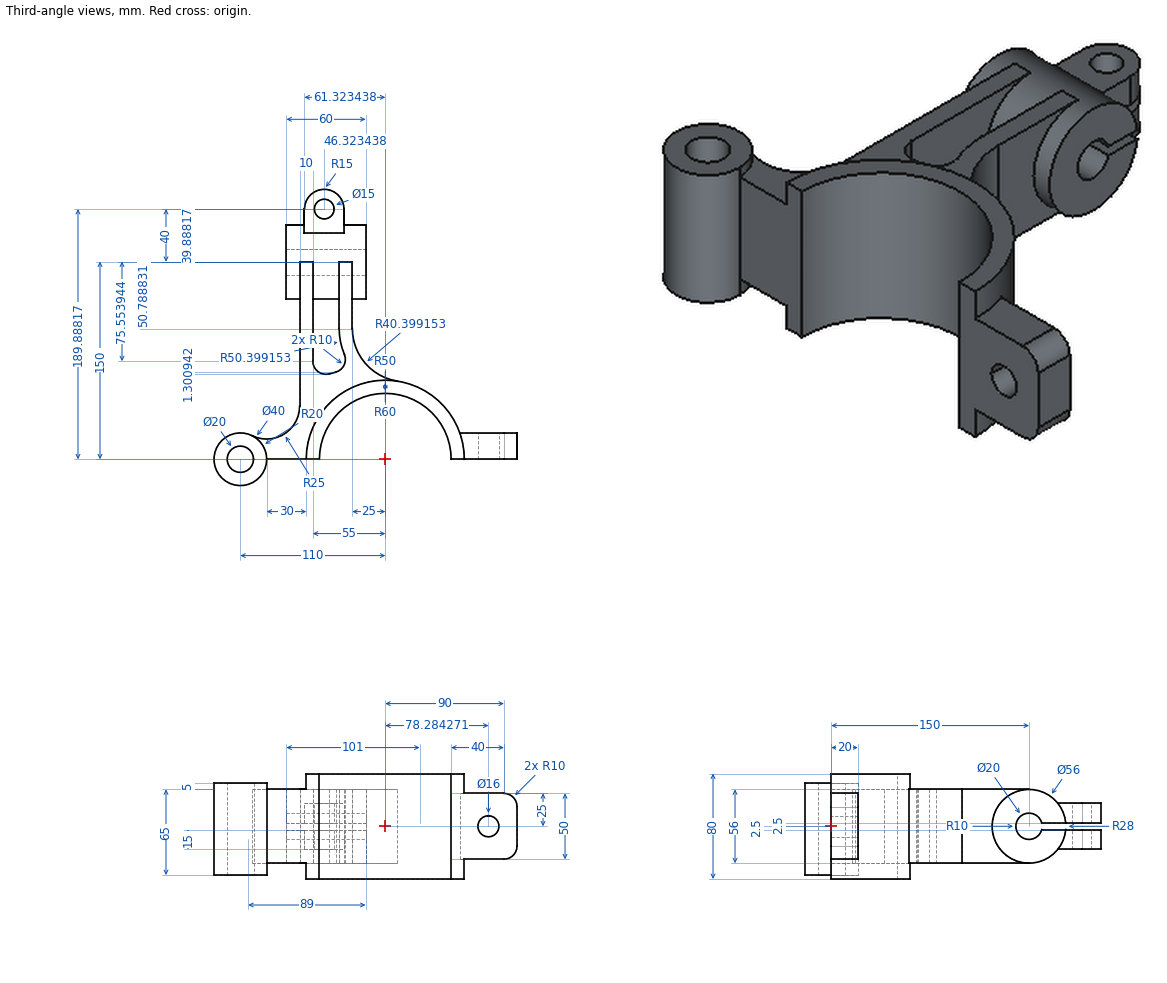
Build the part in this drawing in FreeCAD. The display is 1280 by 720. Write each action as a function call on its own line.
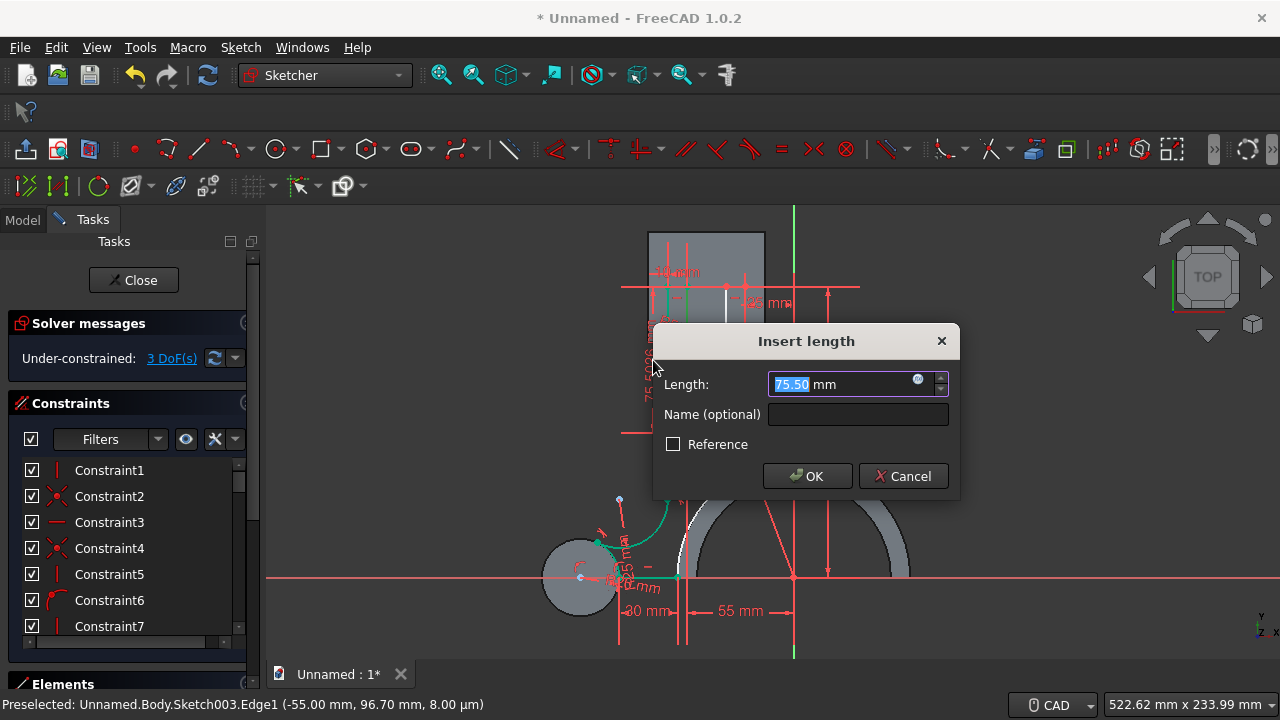
text(75.553944)
key(Return)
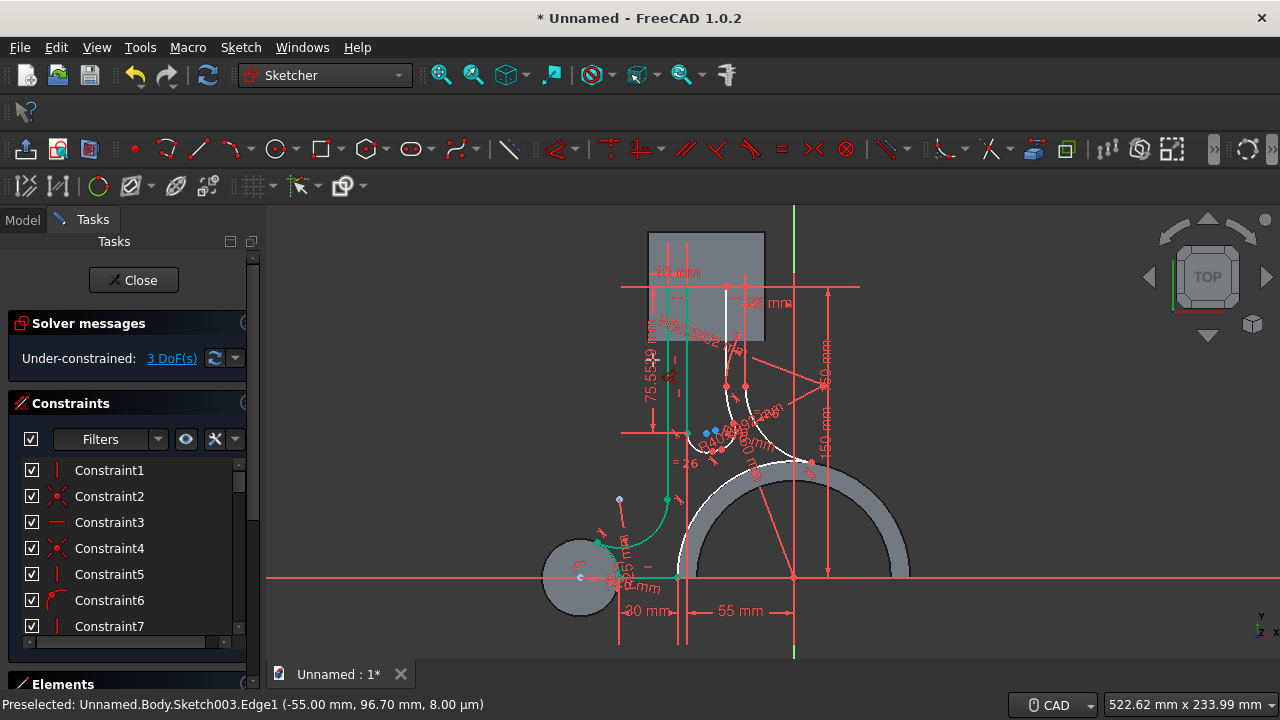
click(745, 357)
click(779, 337)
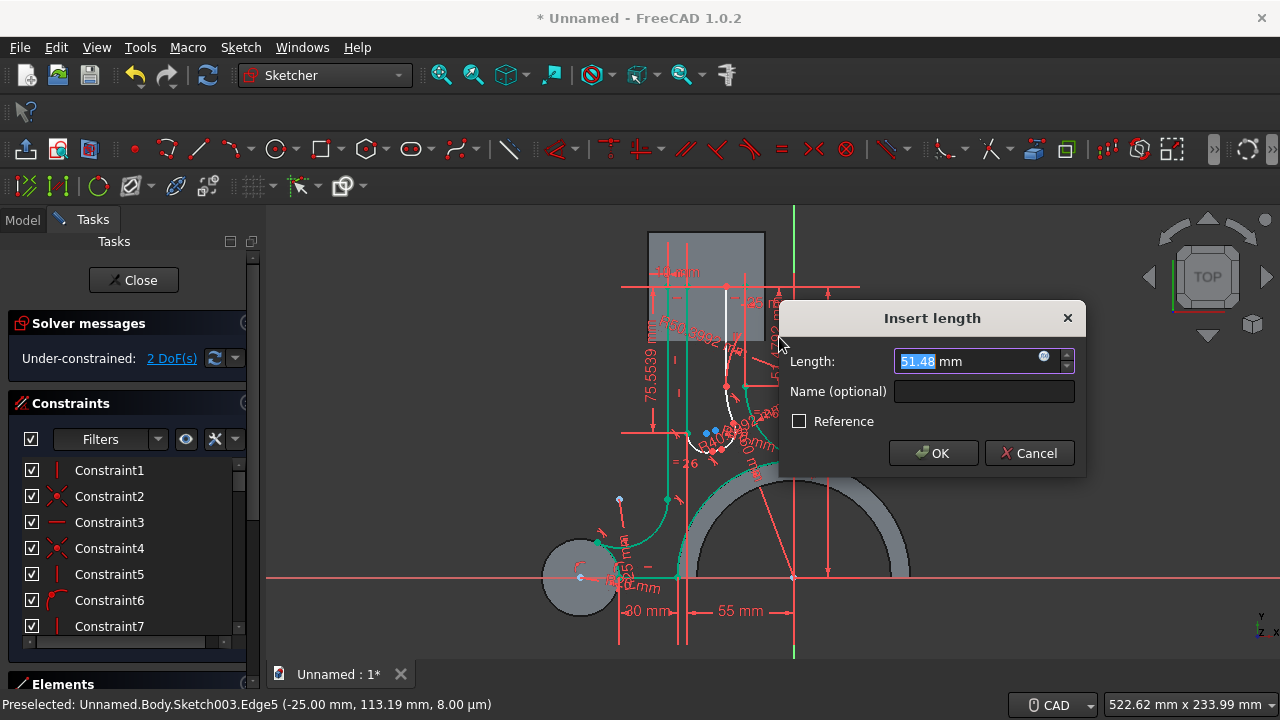
text(50.788831)
key(Return)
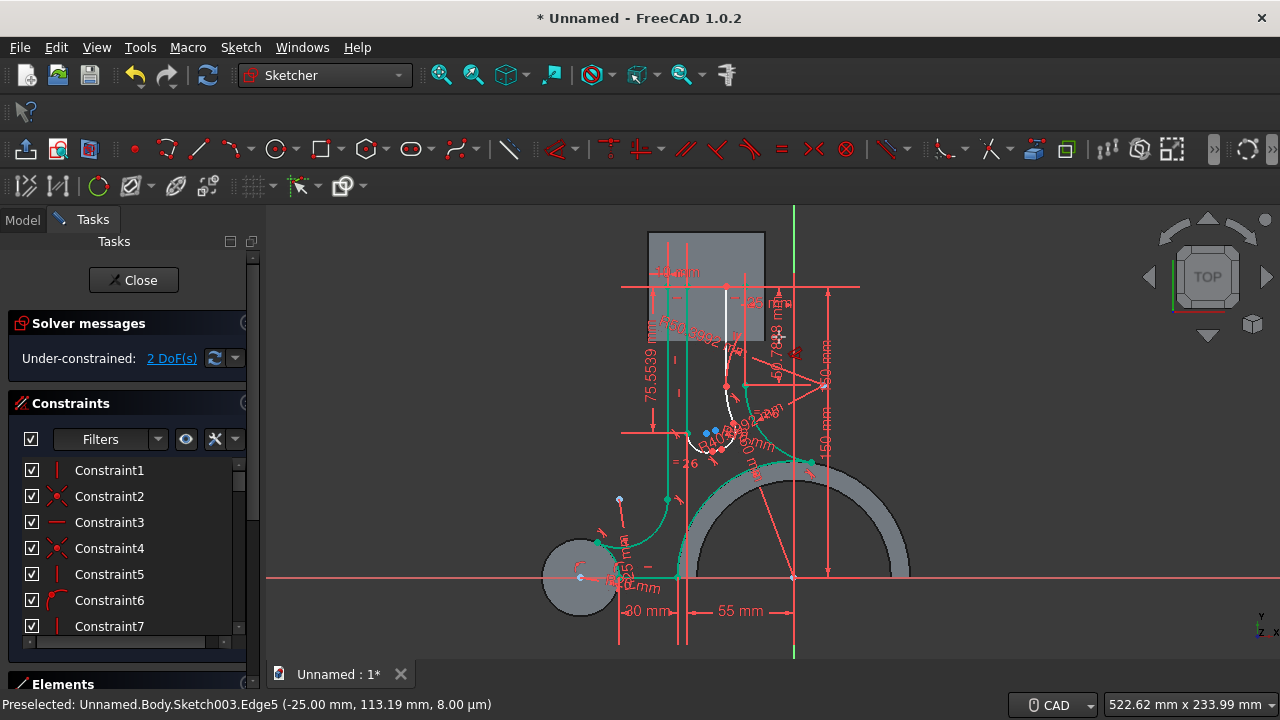
click(726, 317)
click(644, 314)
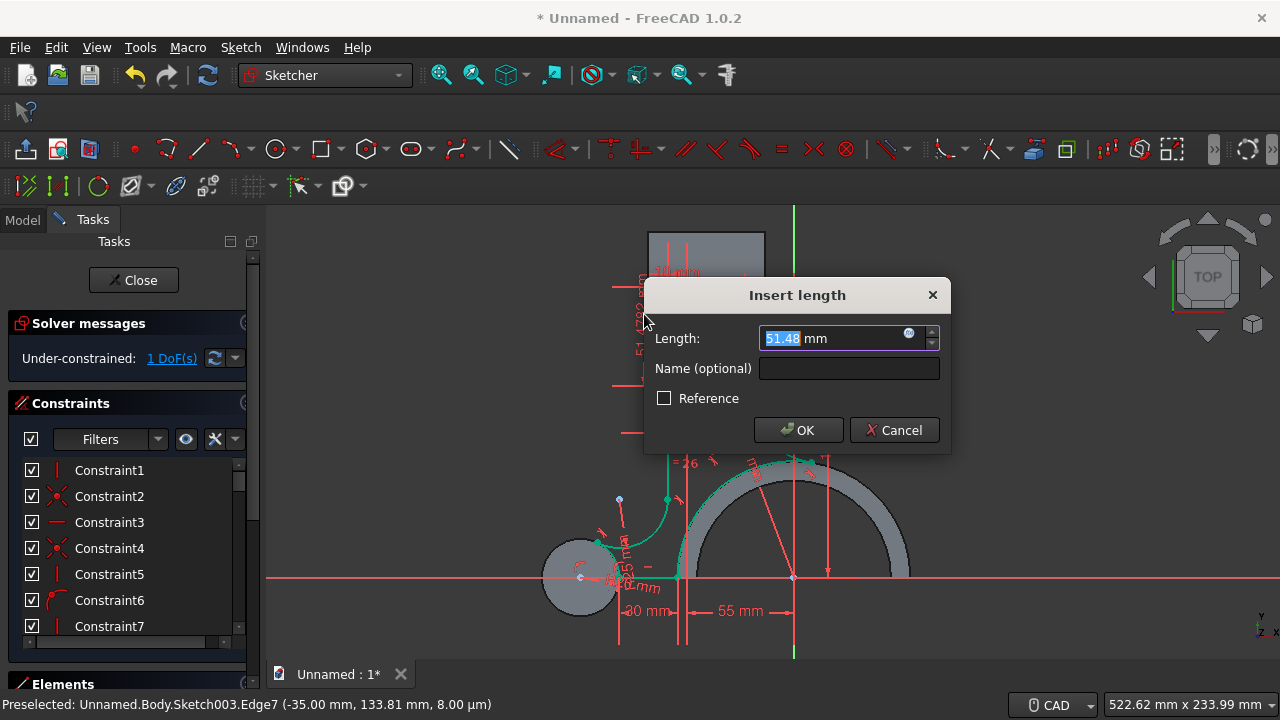
text(50.788831)
key(Return)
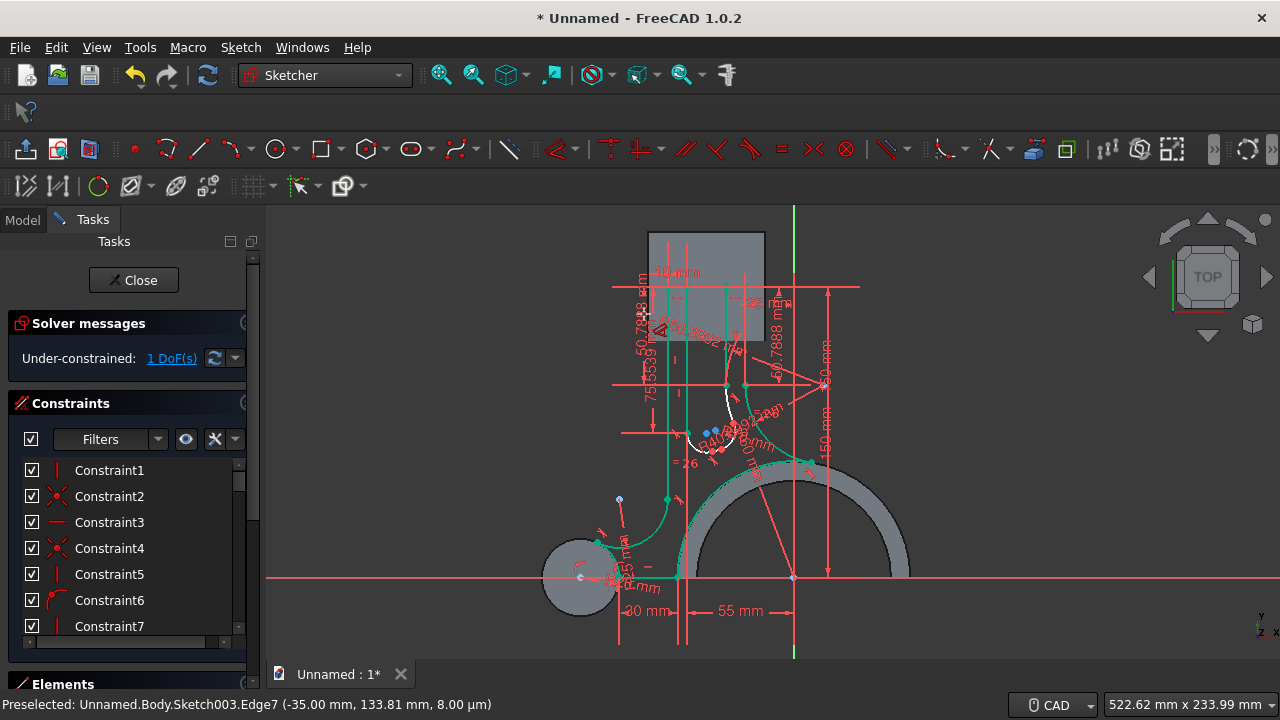
scroll(717, 450, up, 14)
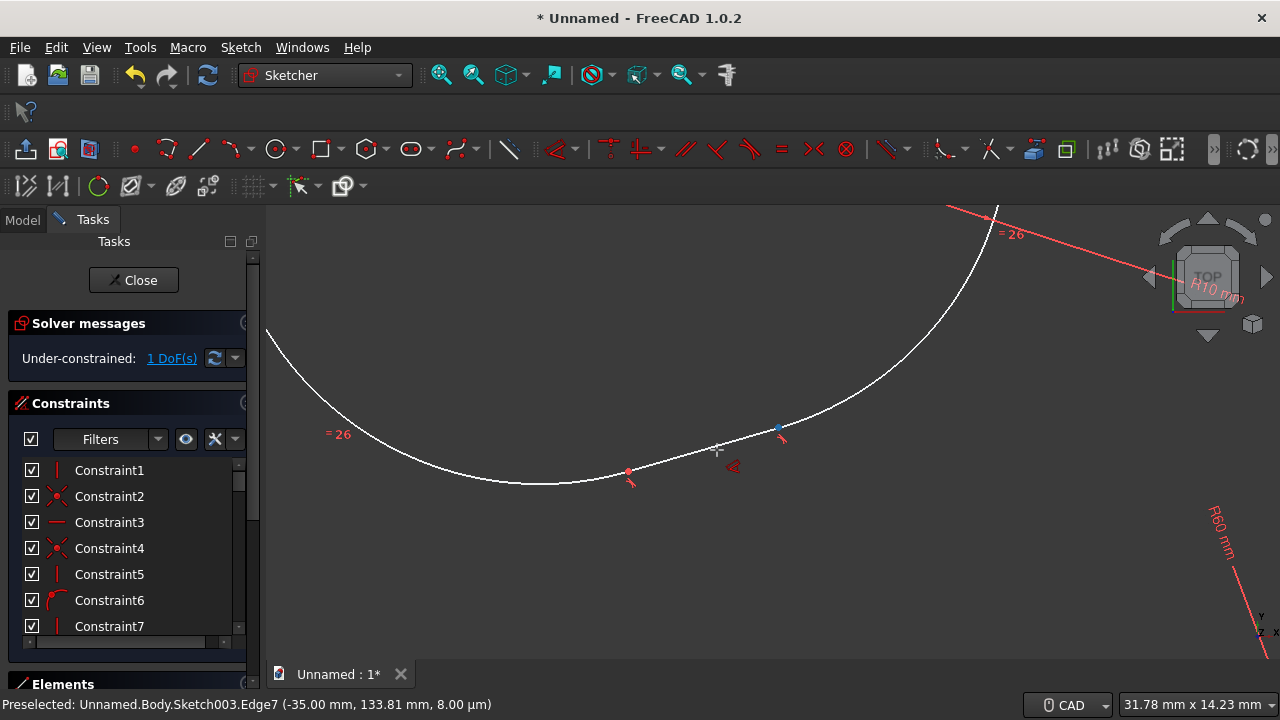
click(704, 450)
click(813, 450)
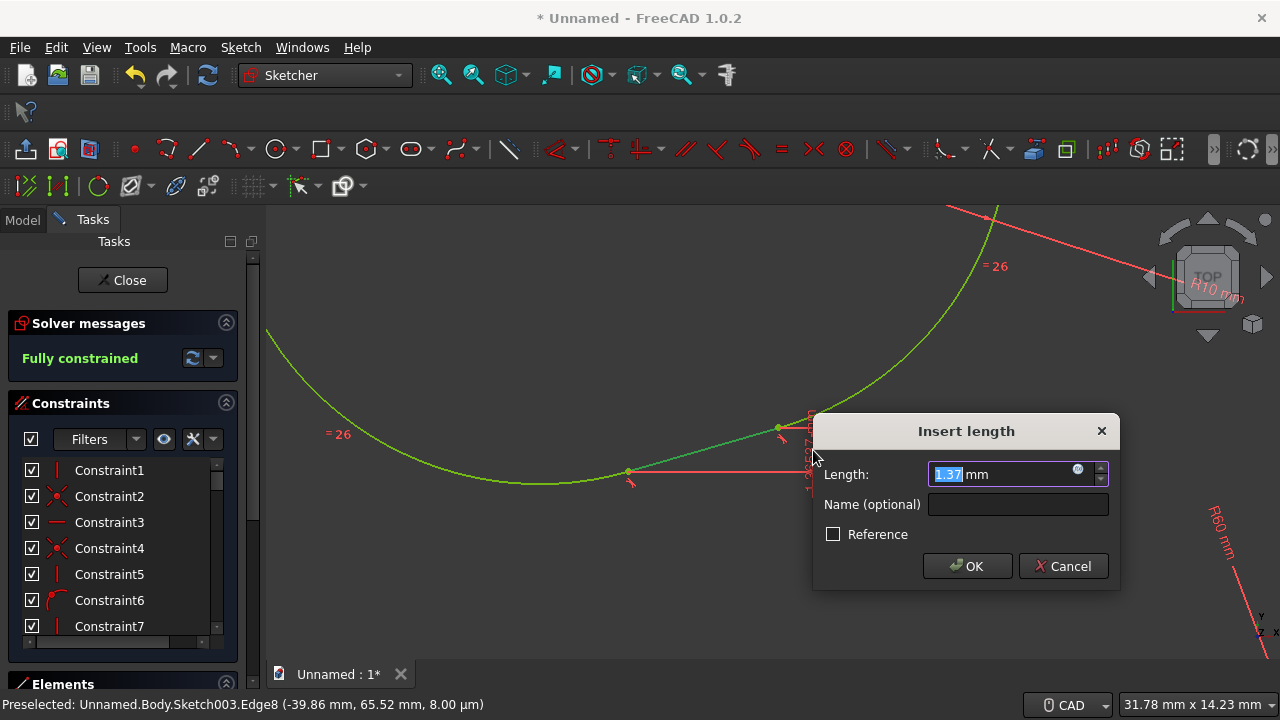
text(1.300942)
key(Return)
key(Escape)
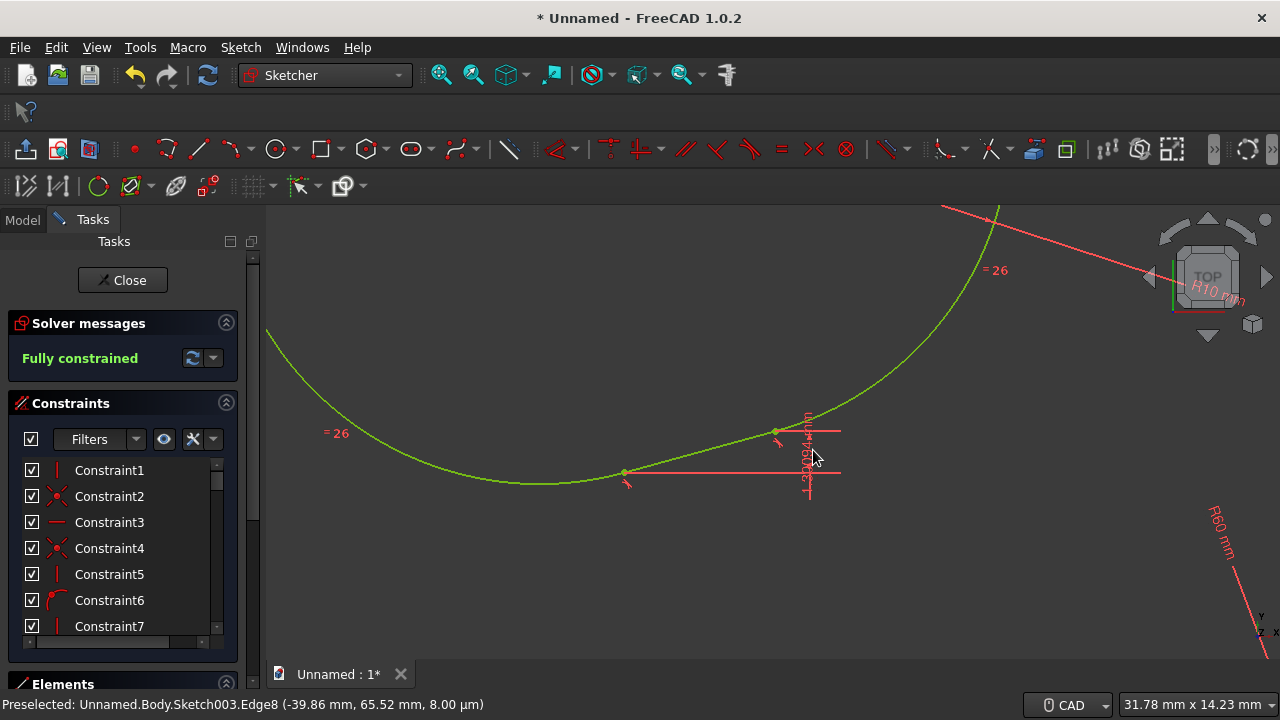
click(123, 280)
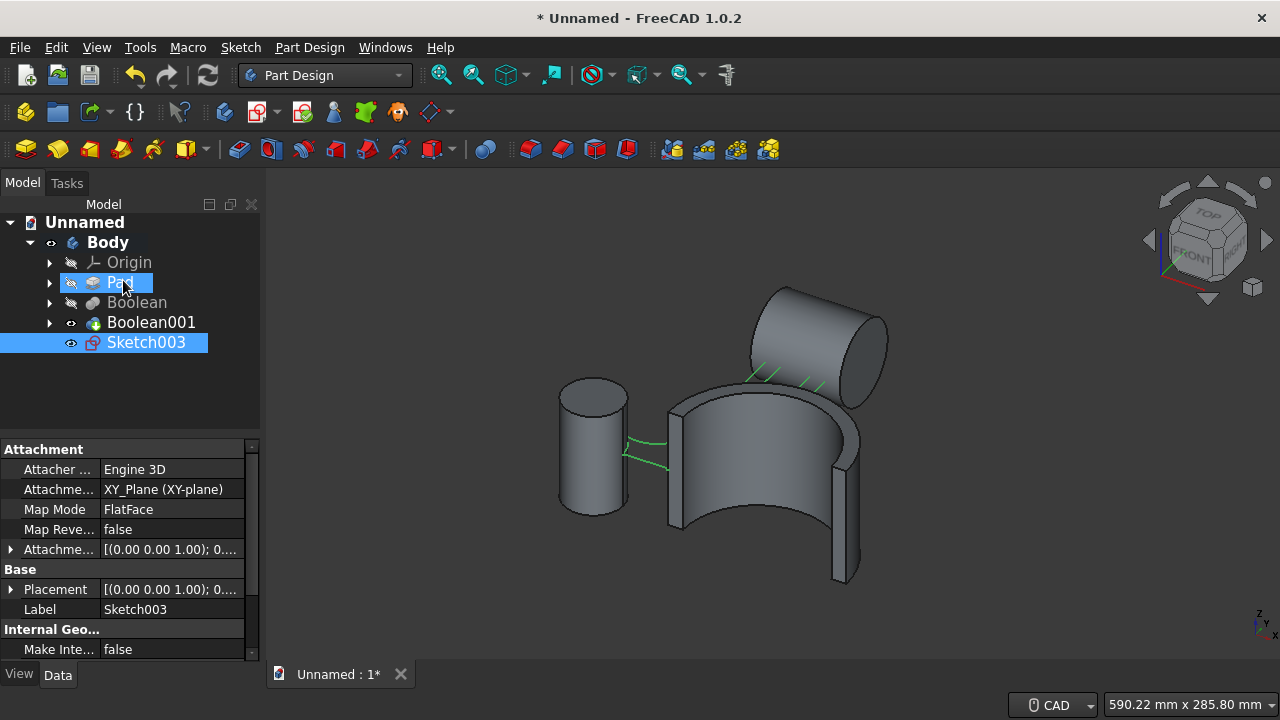
click(26, 150)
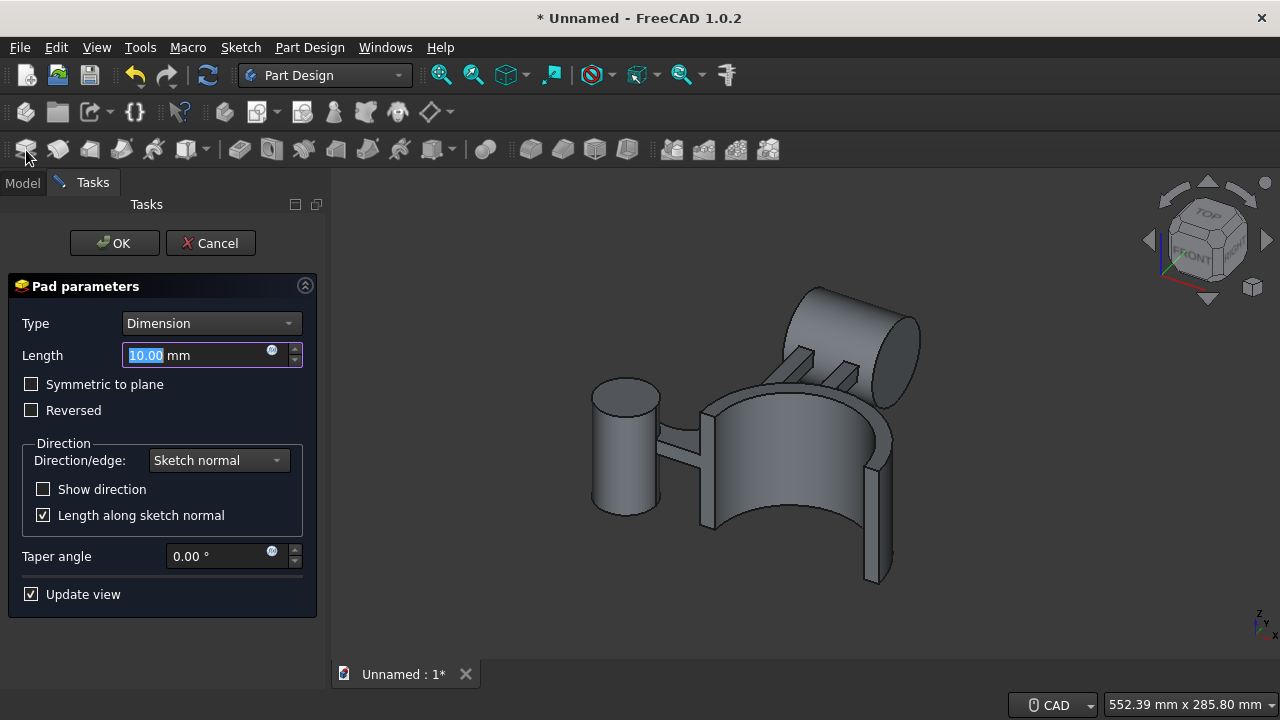
text(56)
key(Tab)